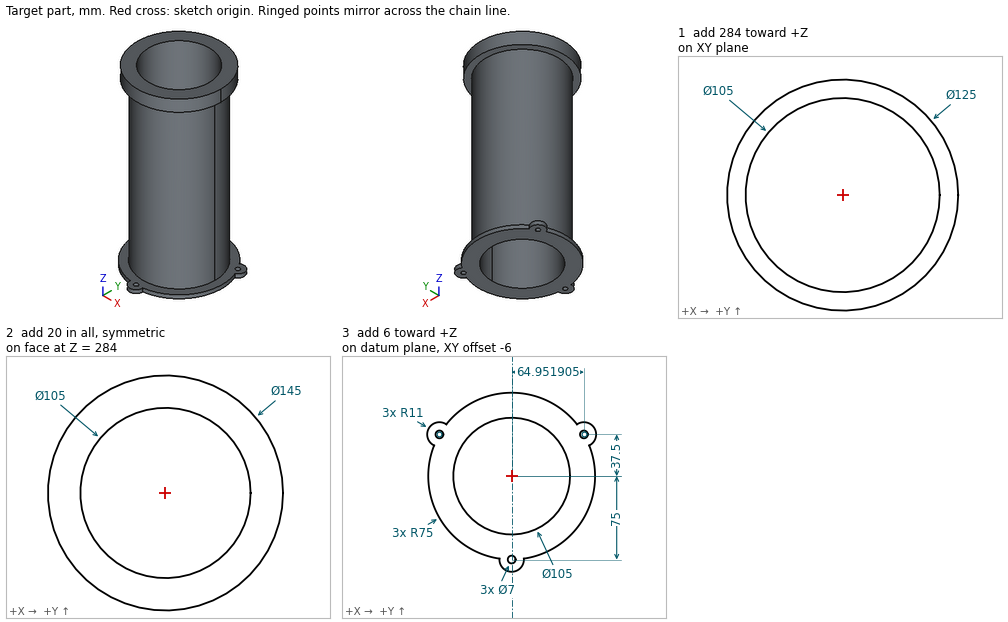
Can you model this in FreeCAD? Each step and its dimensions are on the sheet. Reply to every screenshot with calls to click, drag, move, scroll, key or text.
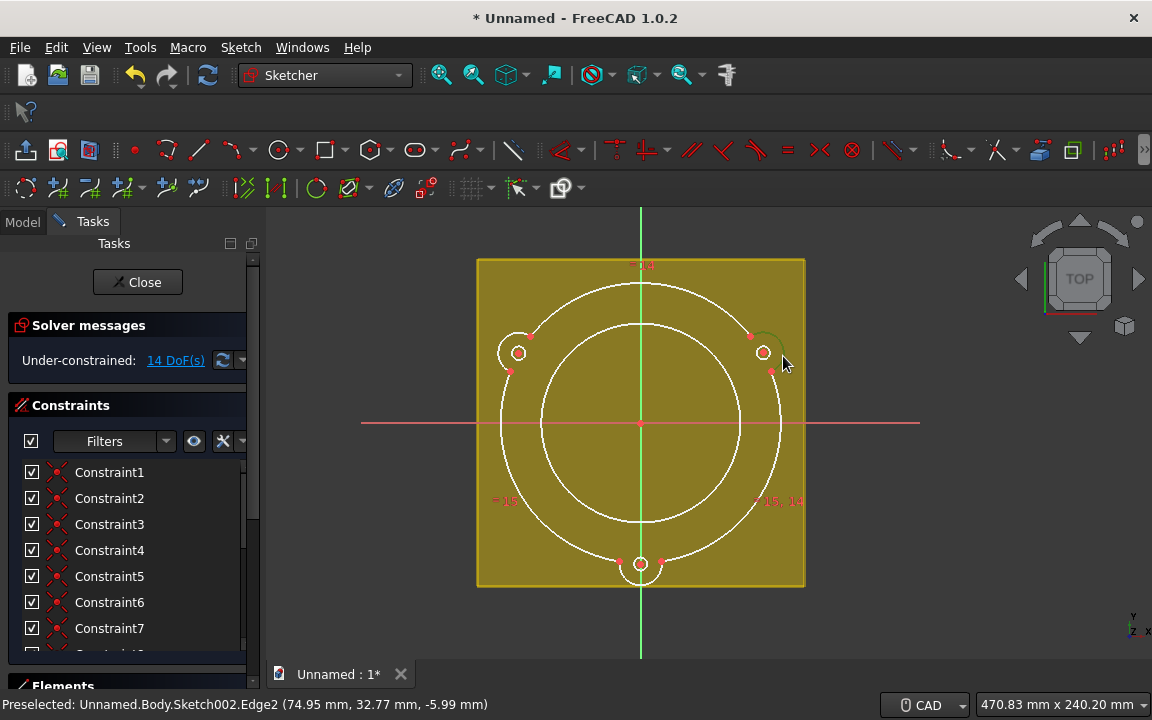
click(627, 581)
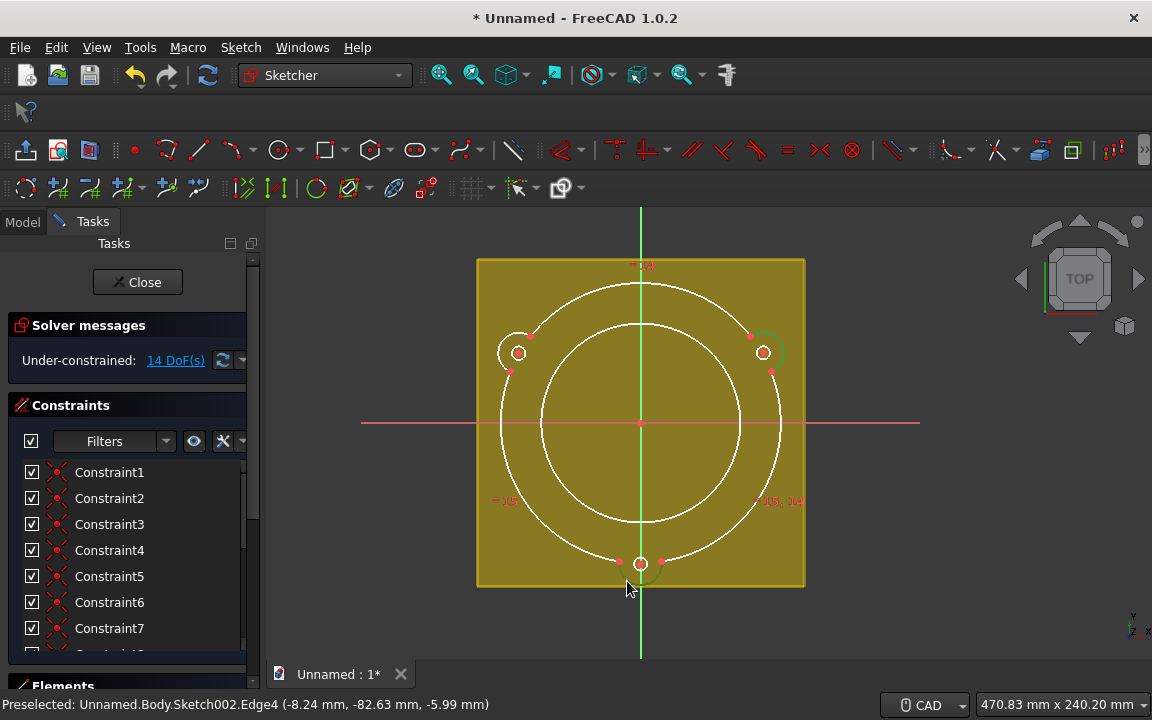
click(511, 334)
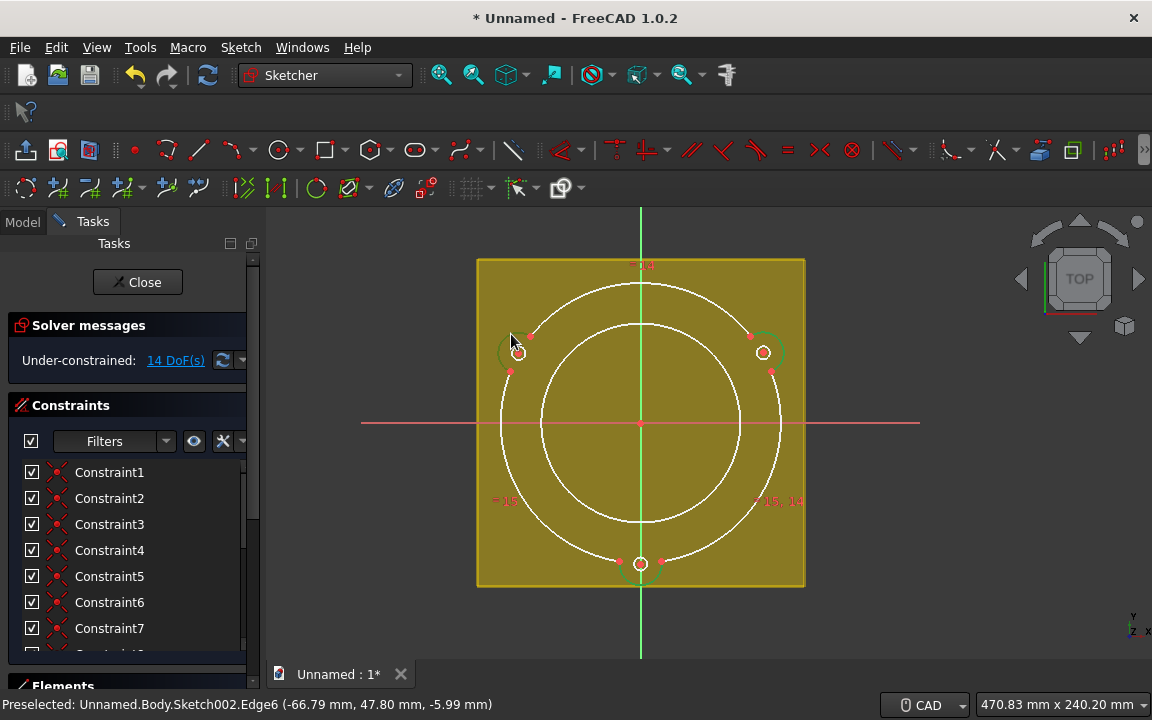
click(788, 150)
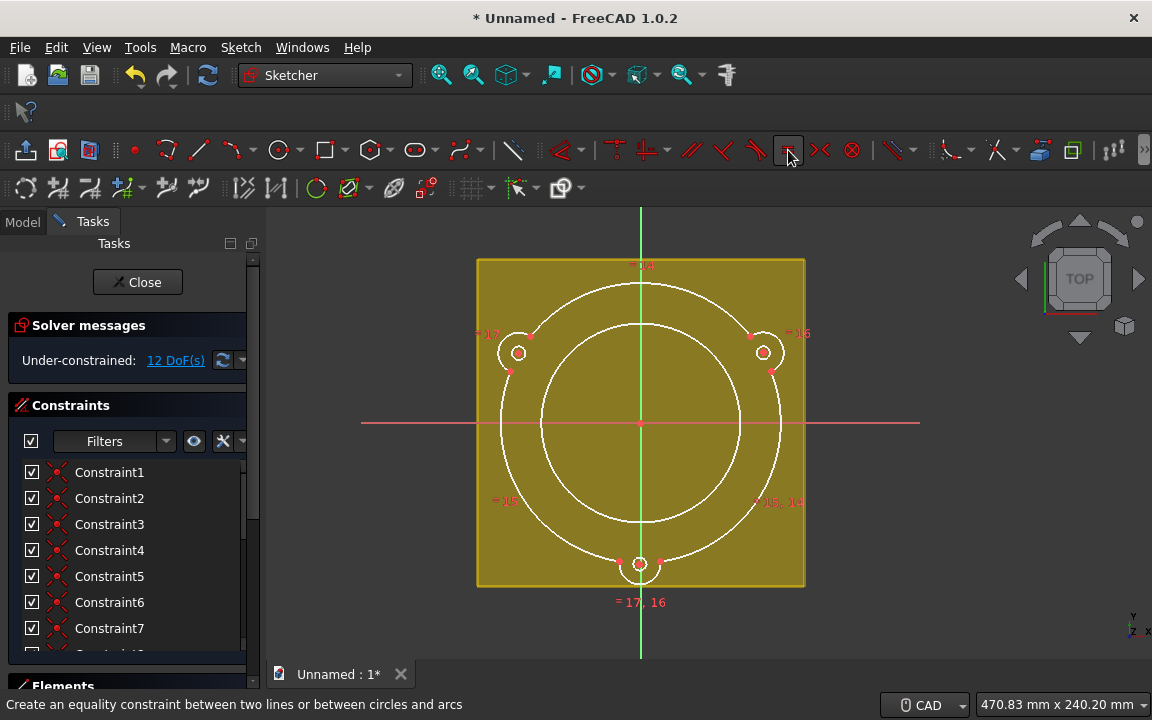
scroll(645, 559, up, 4)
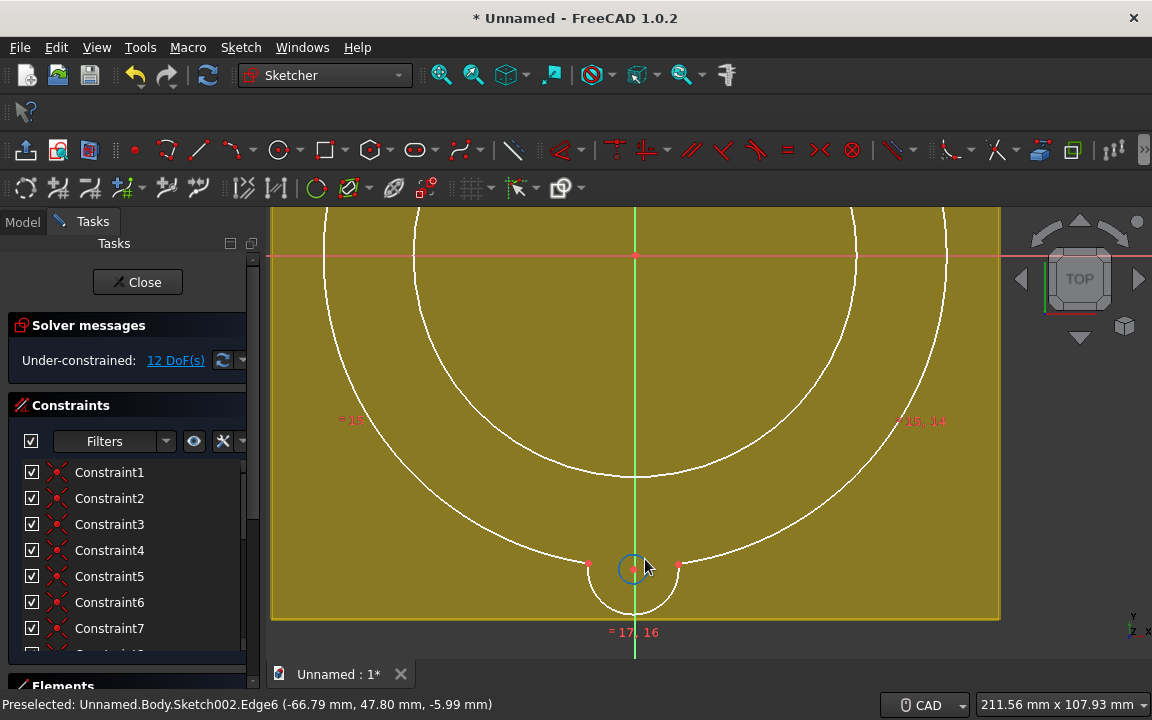
click(643, 559)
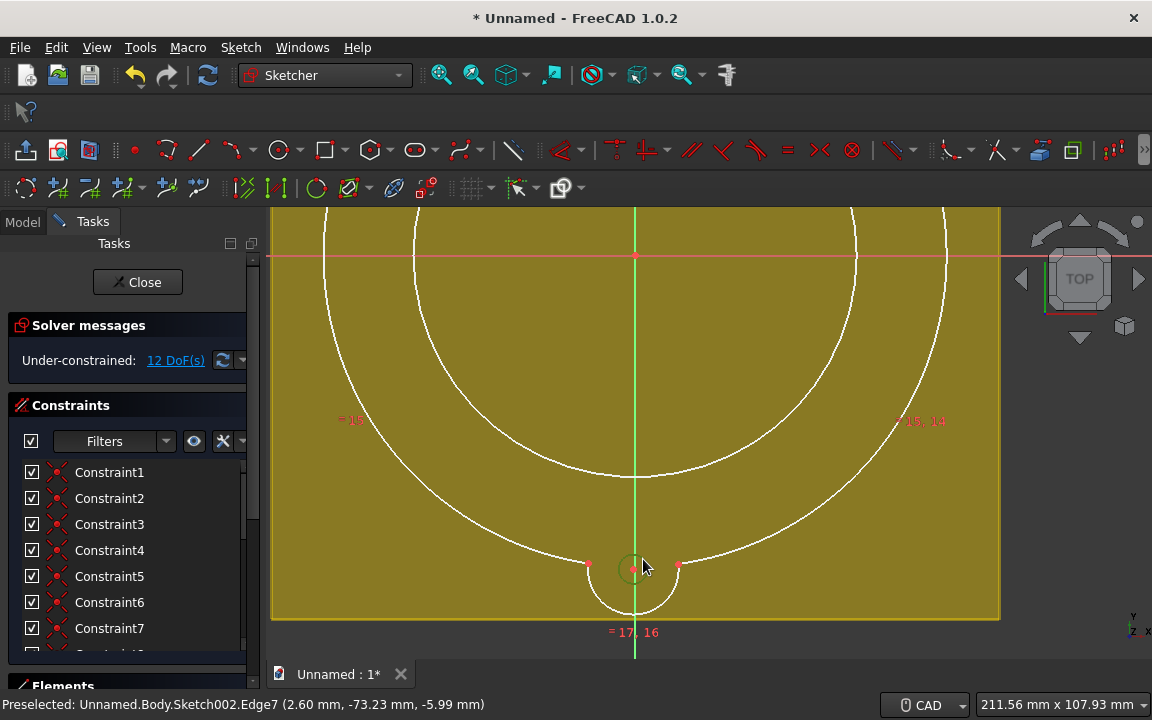
scroll(645, 559, down, 4)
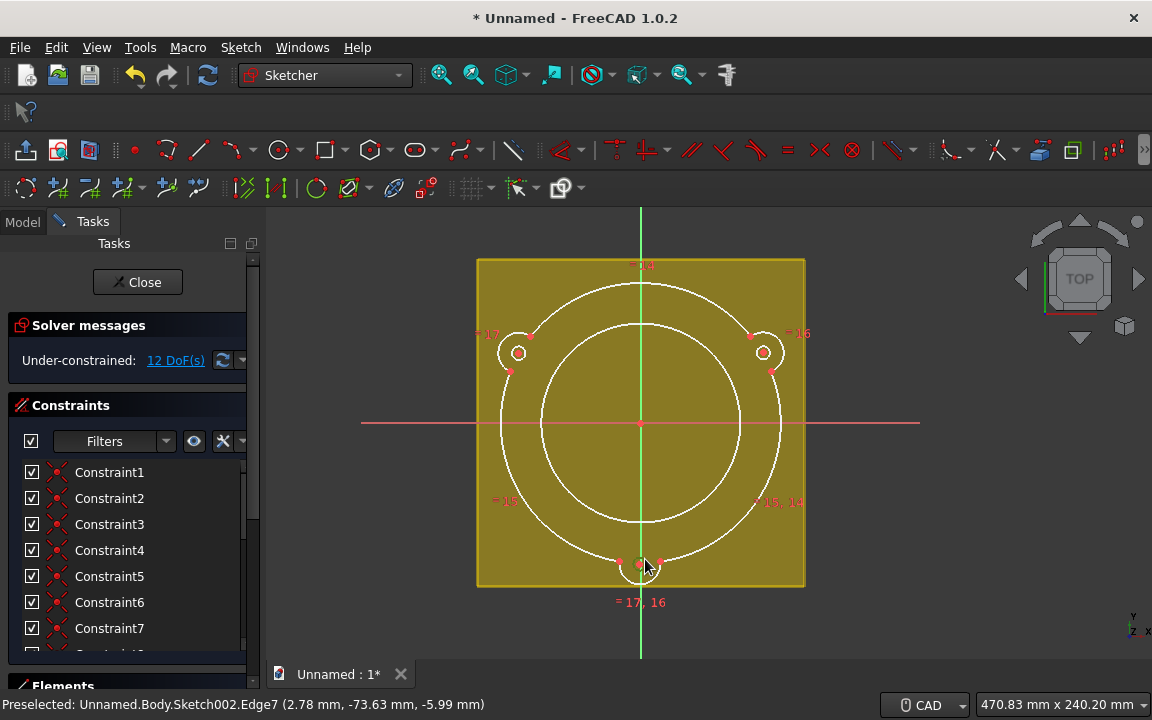
scroll(768, 348, up, 4)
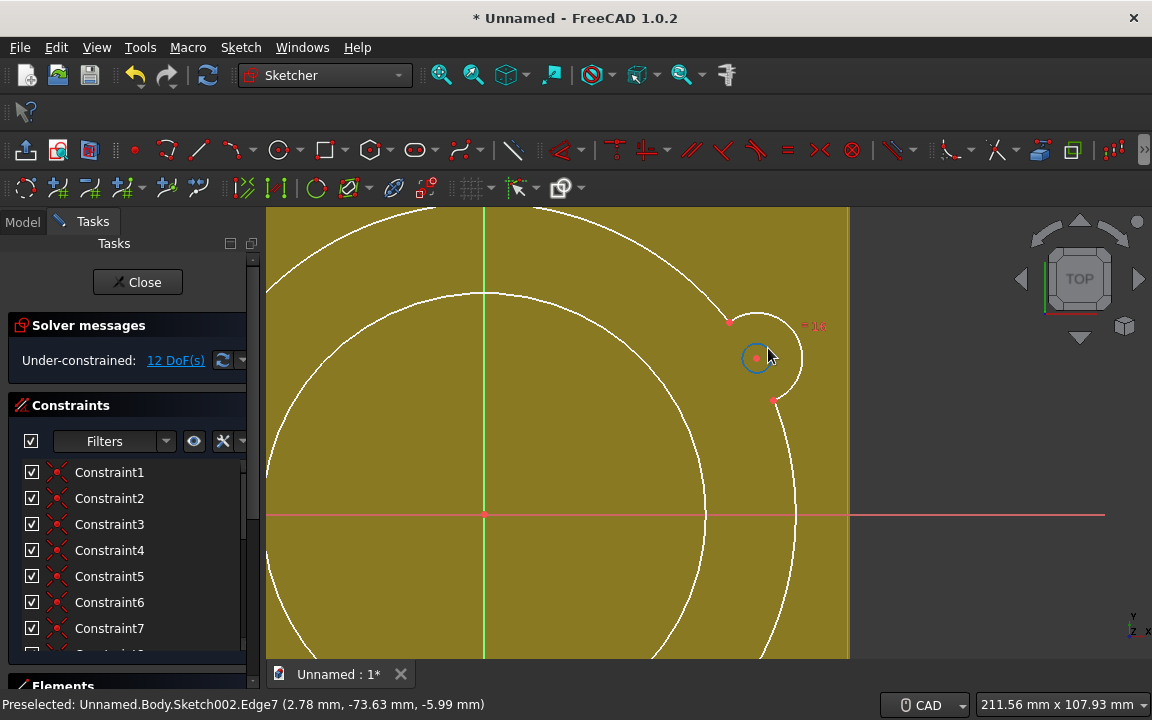
click(767, 348)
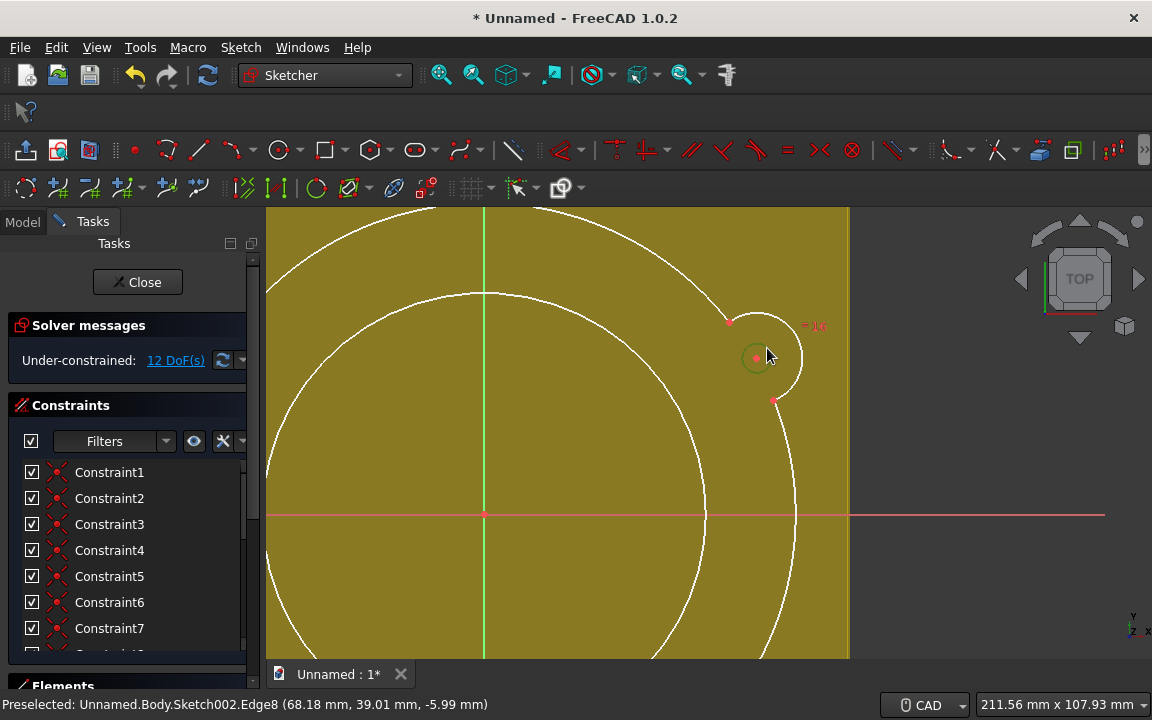
scroll(768, 348, down, 4)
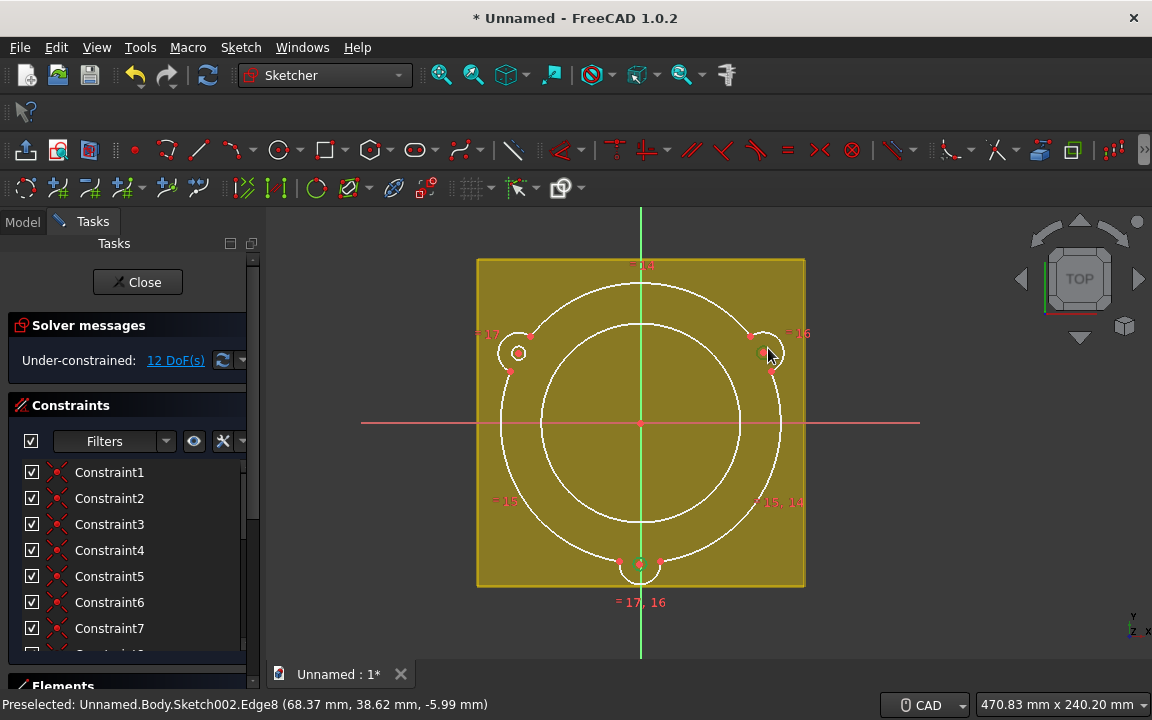
scroll(523, 348, up, 4)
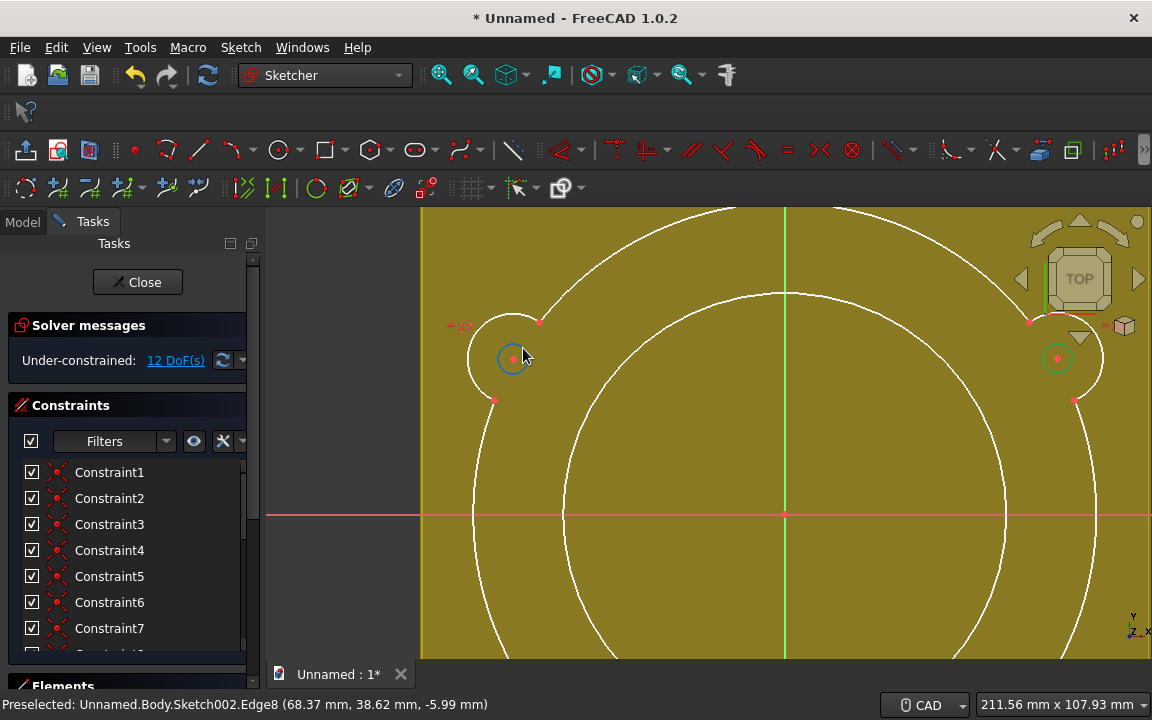
click(524, 349)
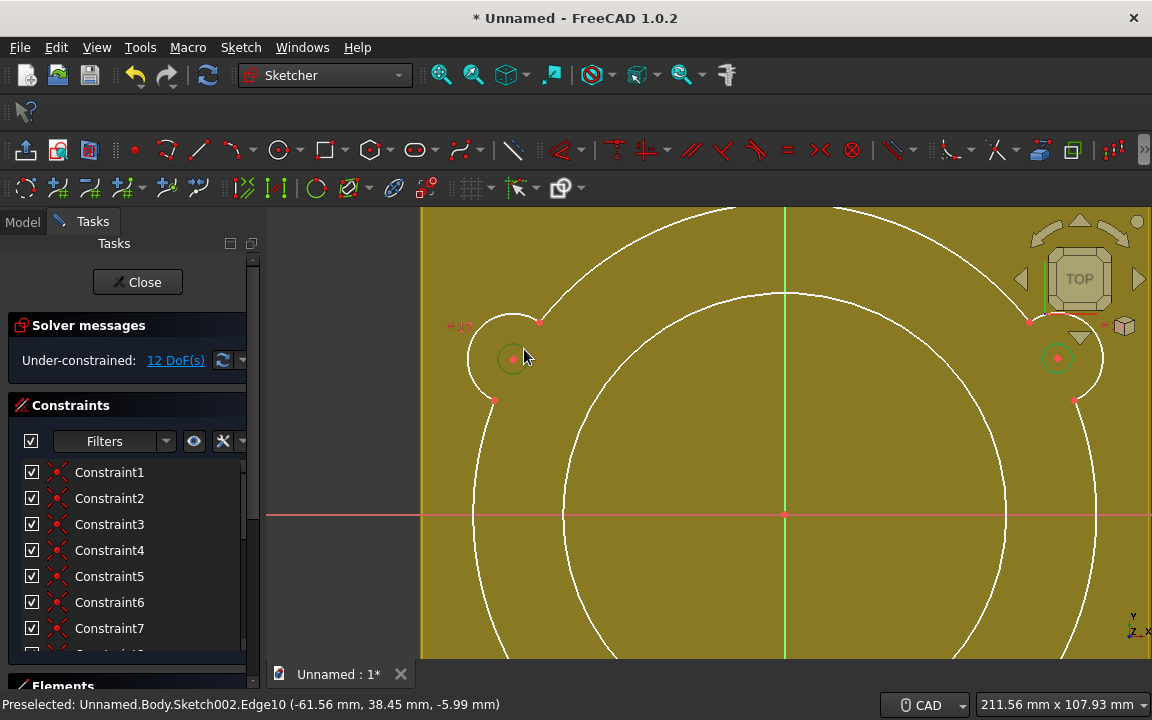
click(788, 150)